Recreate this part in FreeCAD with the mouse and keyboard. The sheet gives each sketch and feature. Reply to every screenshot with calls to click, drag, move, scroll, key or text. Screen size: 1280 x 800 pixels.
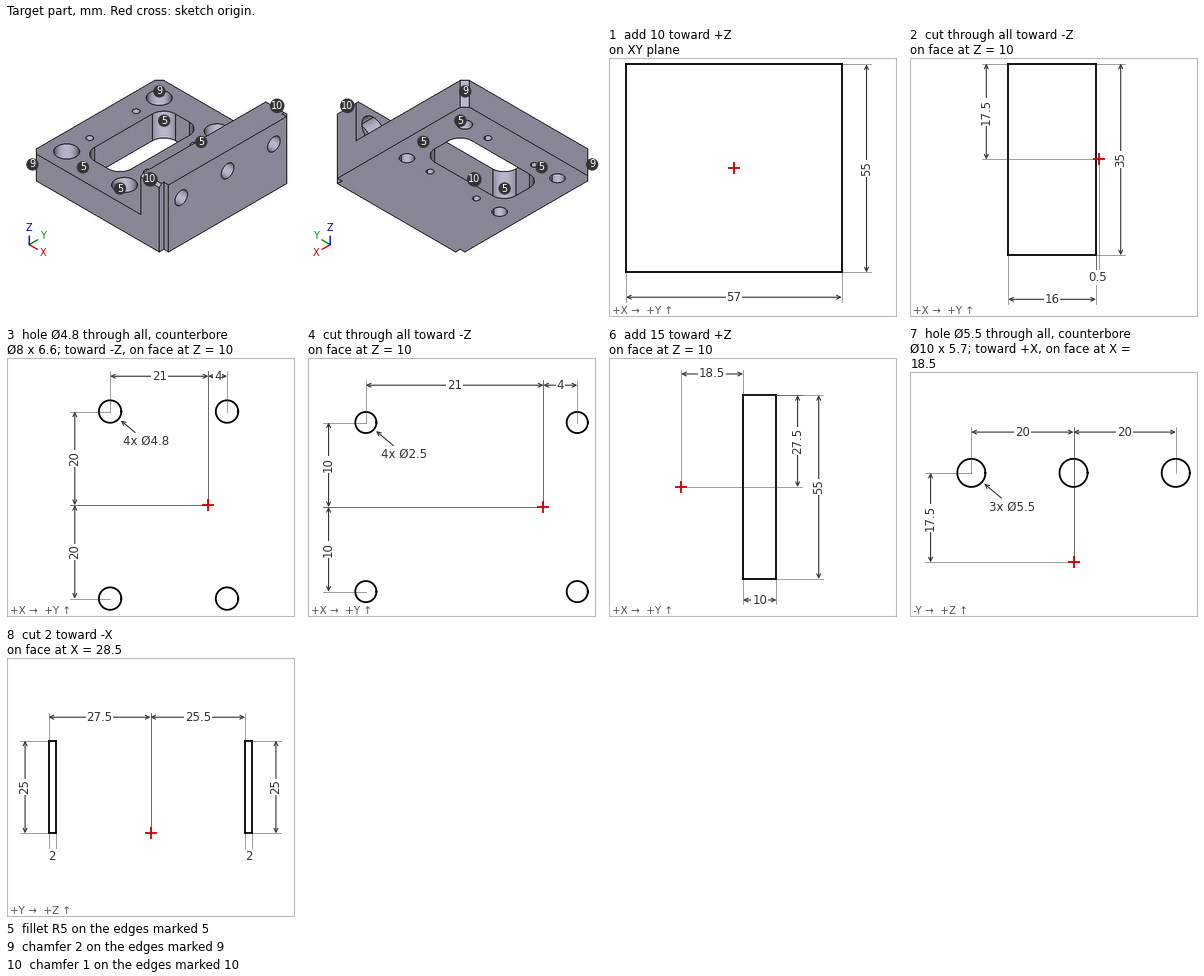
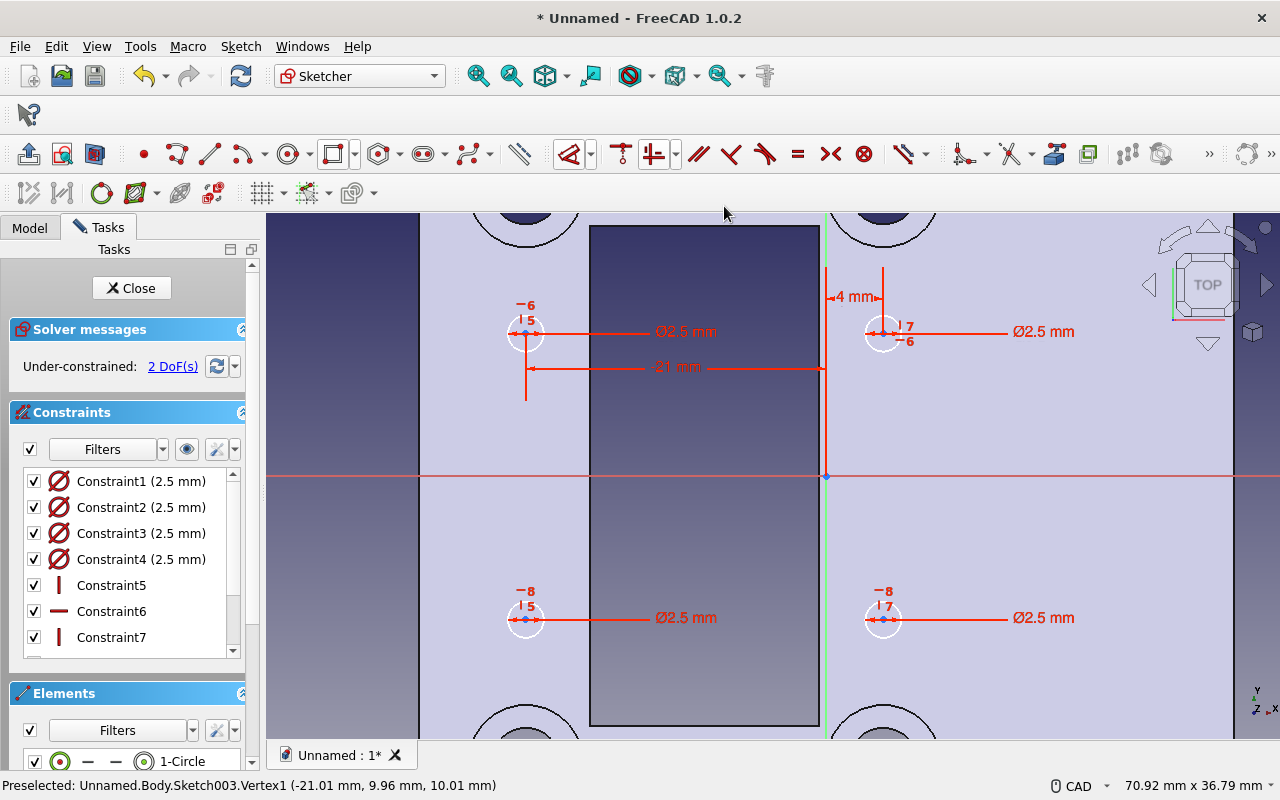
click(526, 334)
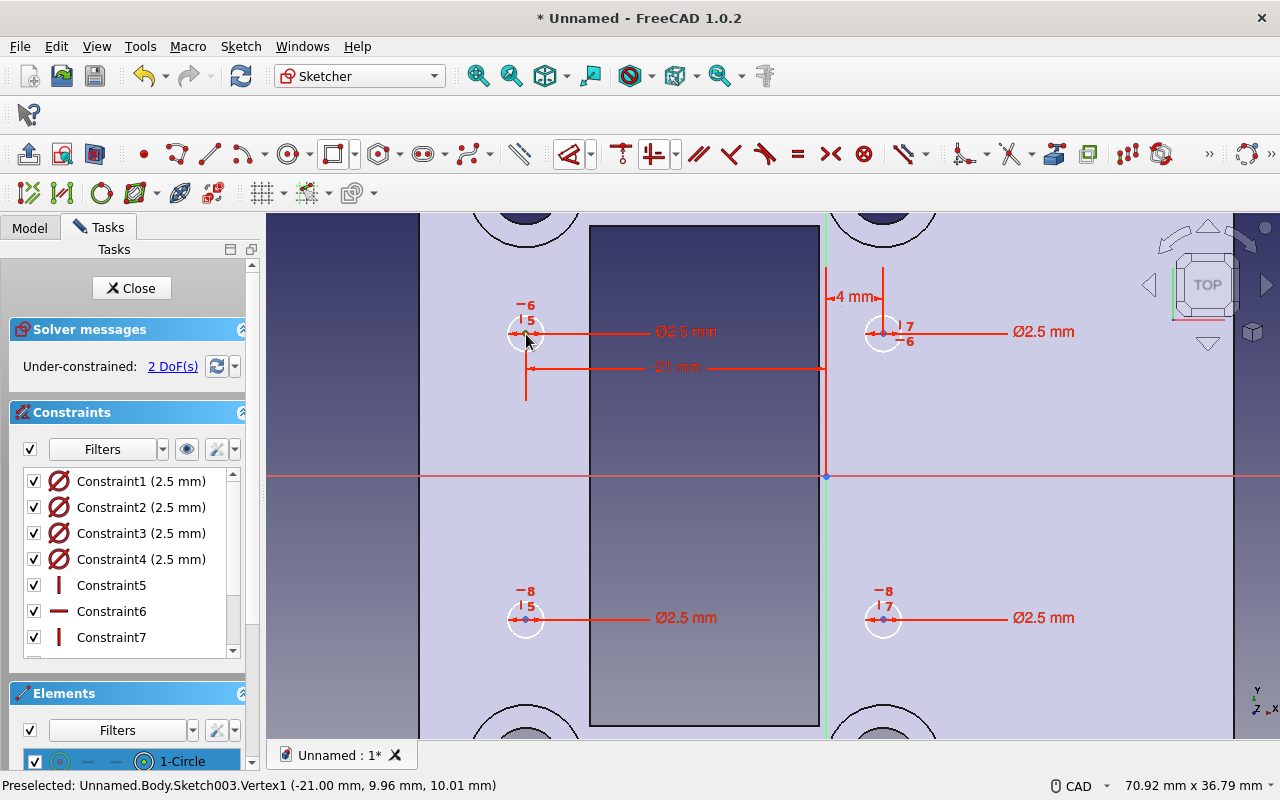
key(i)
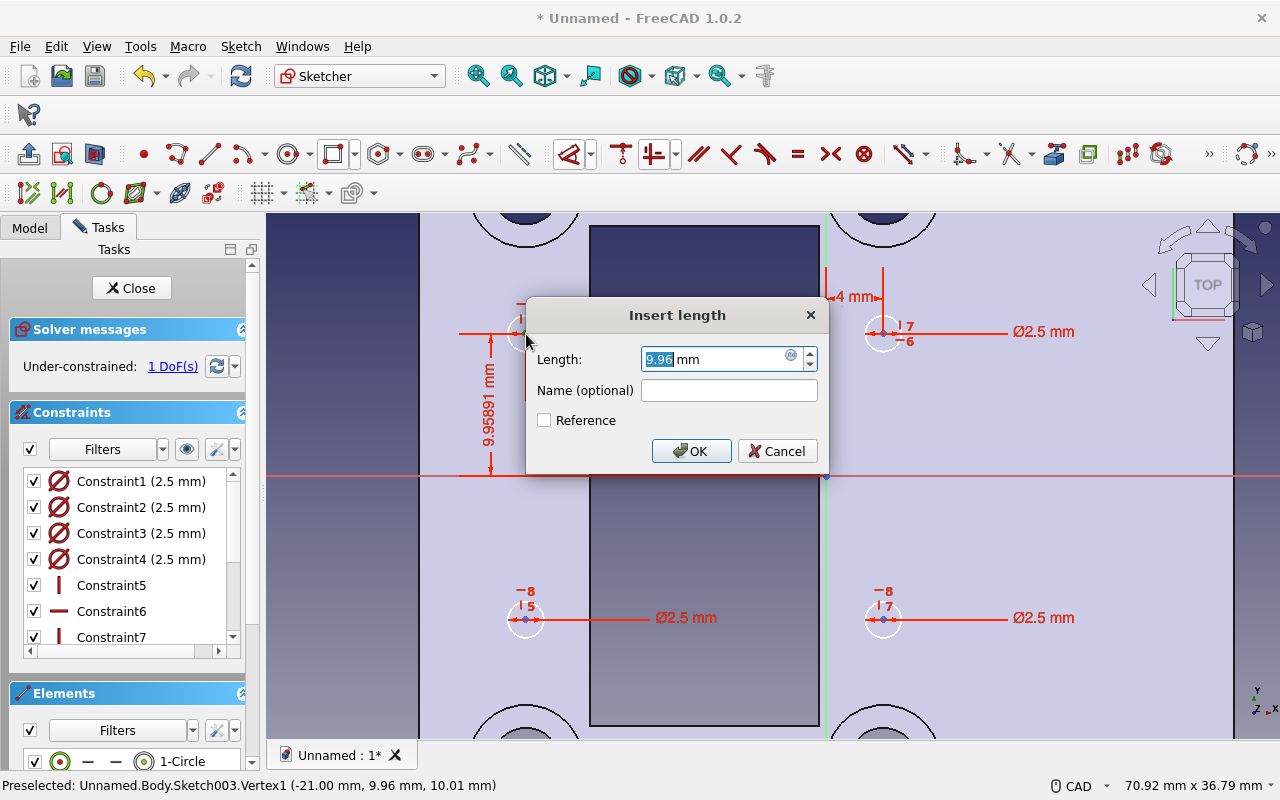
text(10)
key(Return)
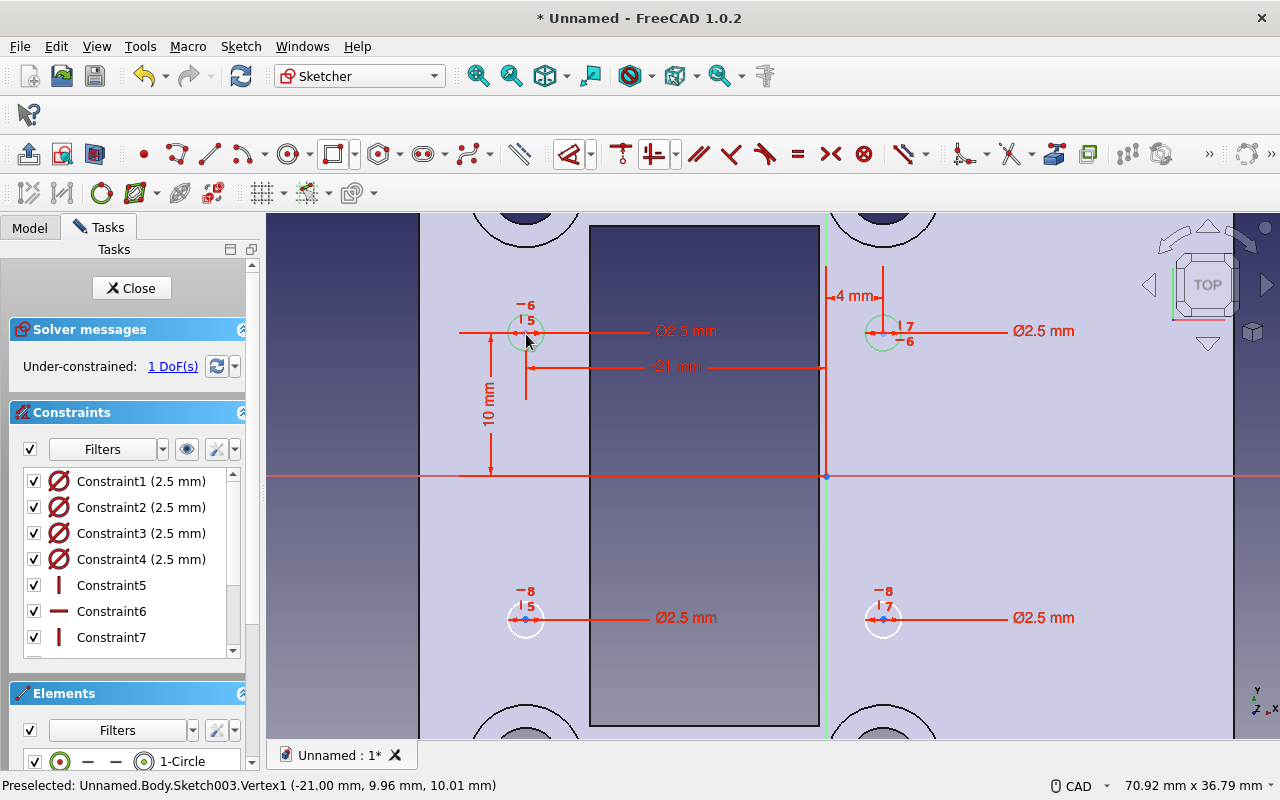
click(526, 620)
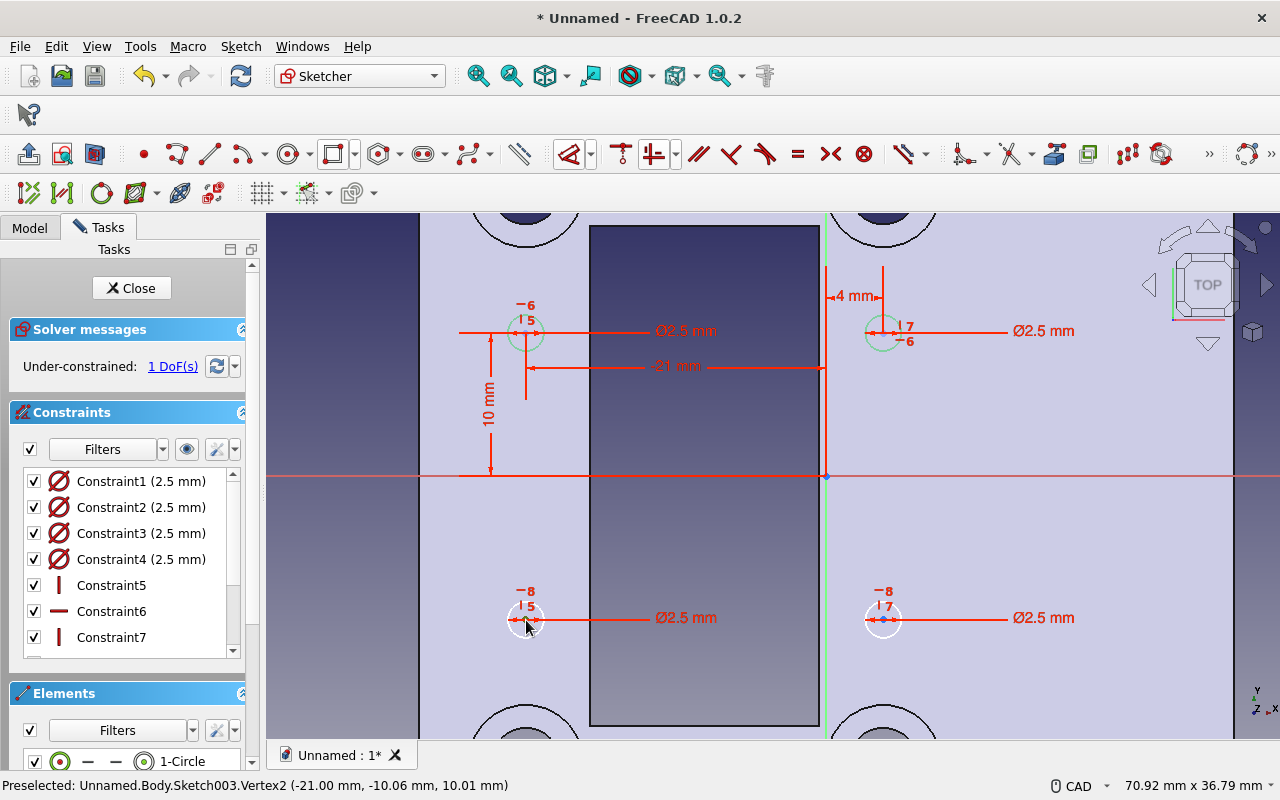
click(590, 154)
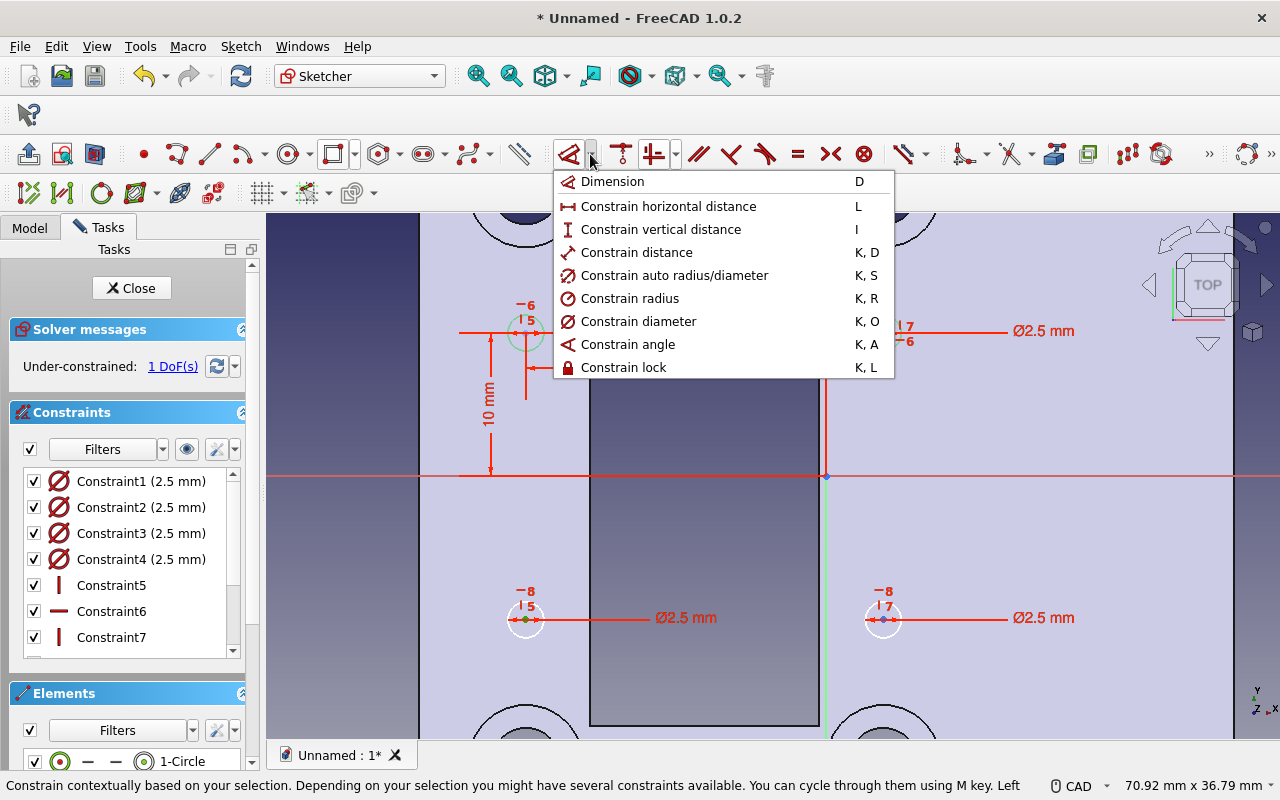
click(724, 230)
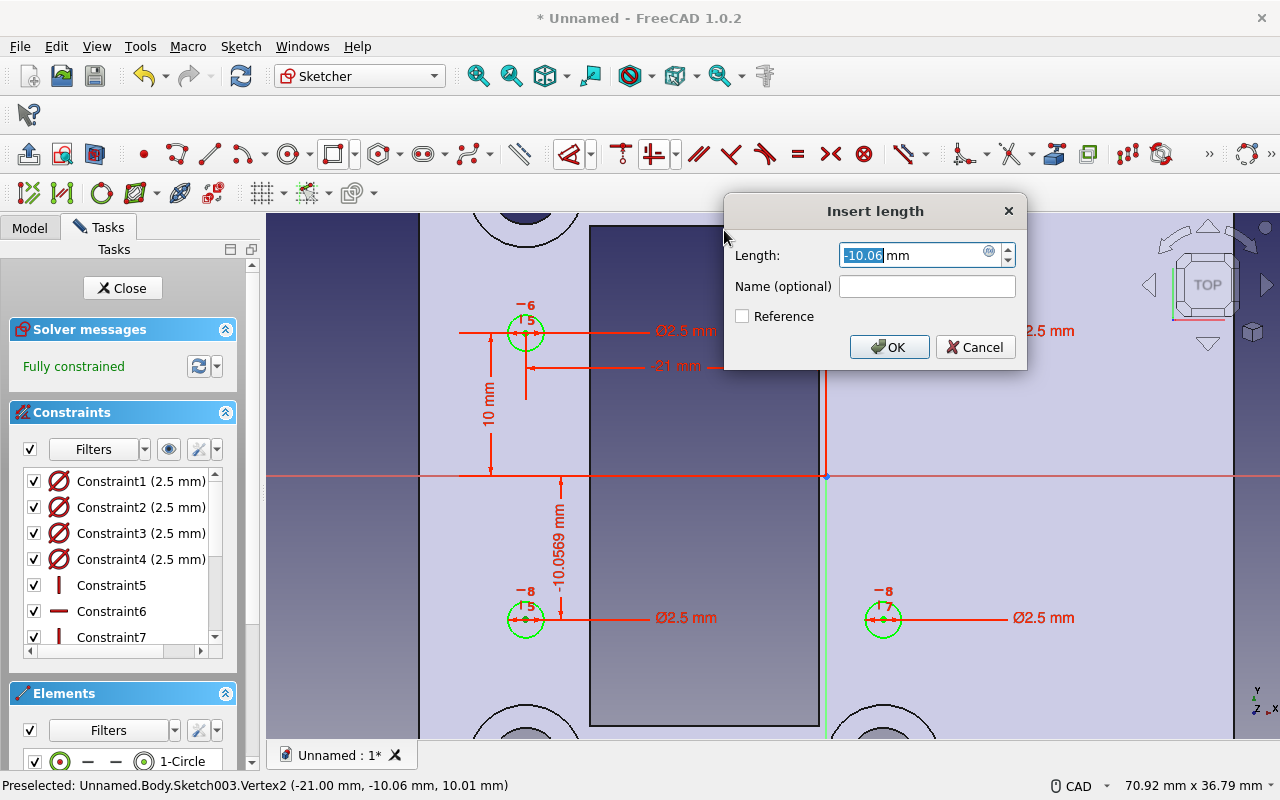
text(-10)
key(Return)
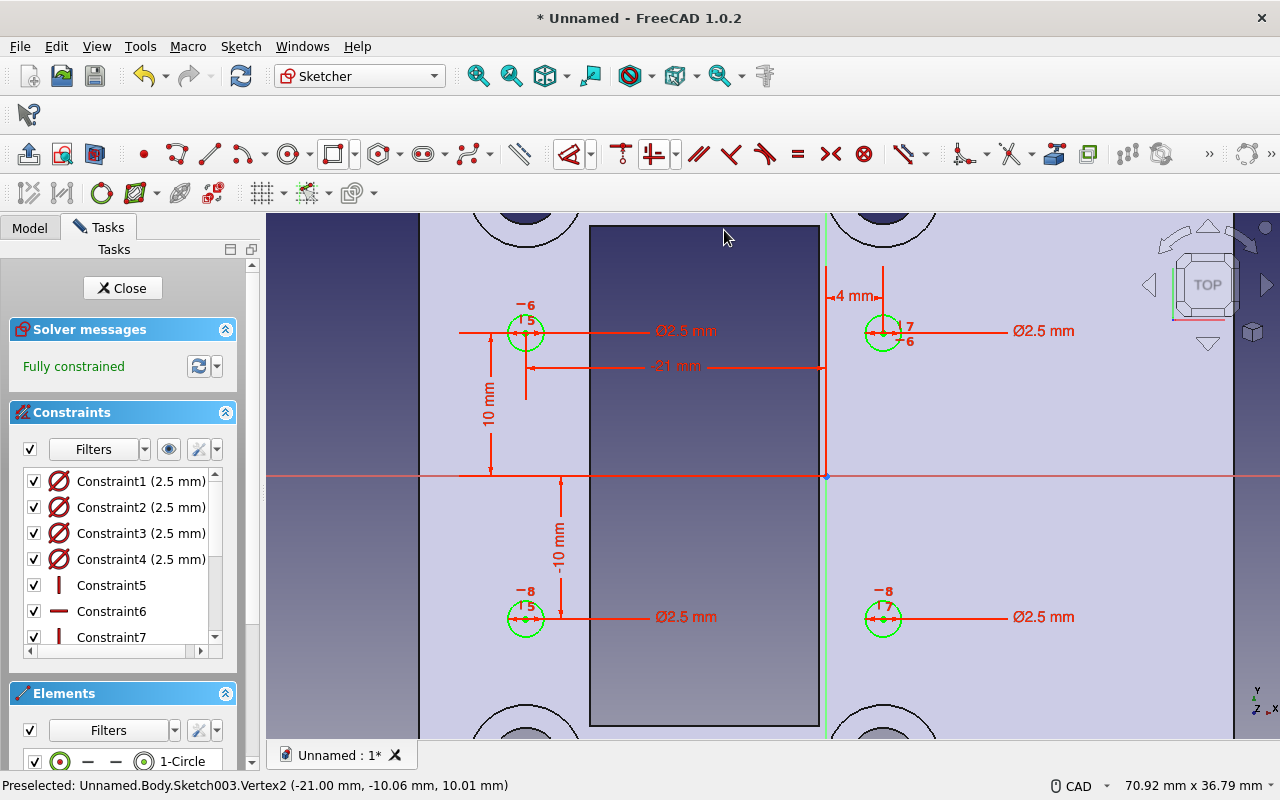
click(123, 288)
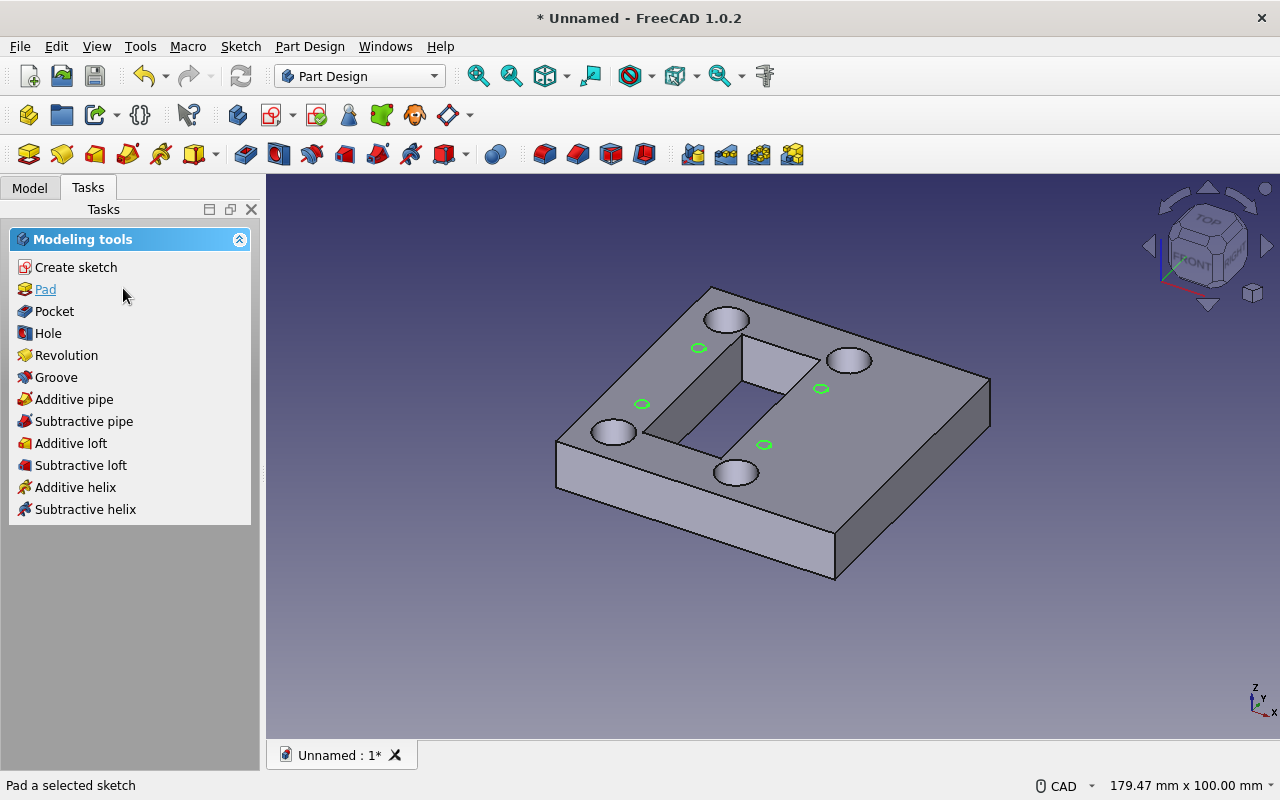
click(246, 154)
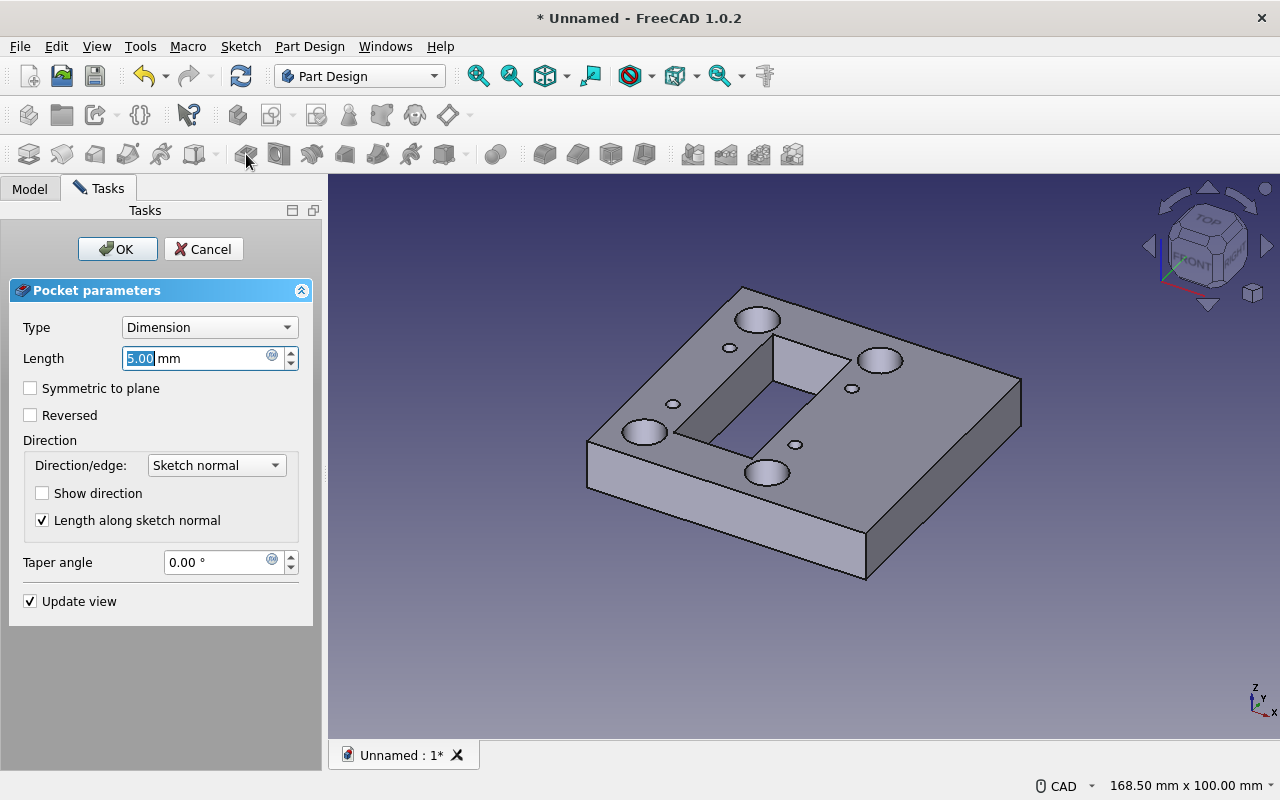
click(210, 328)